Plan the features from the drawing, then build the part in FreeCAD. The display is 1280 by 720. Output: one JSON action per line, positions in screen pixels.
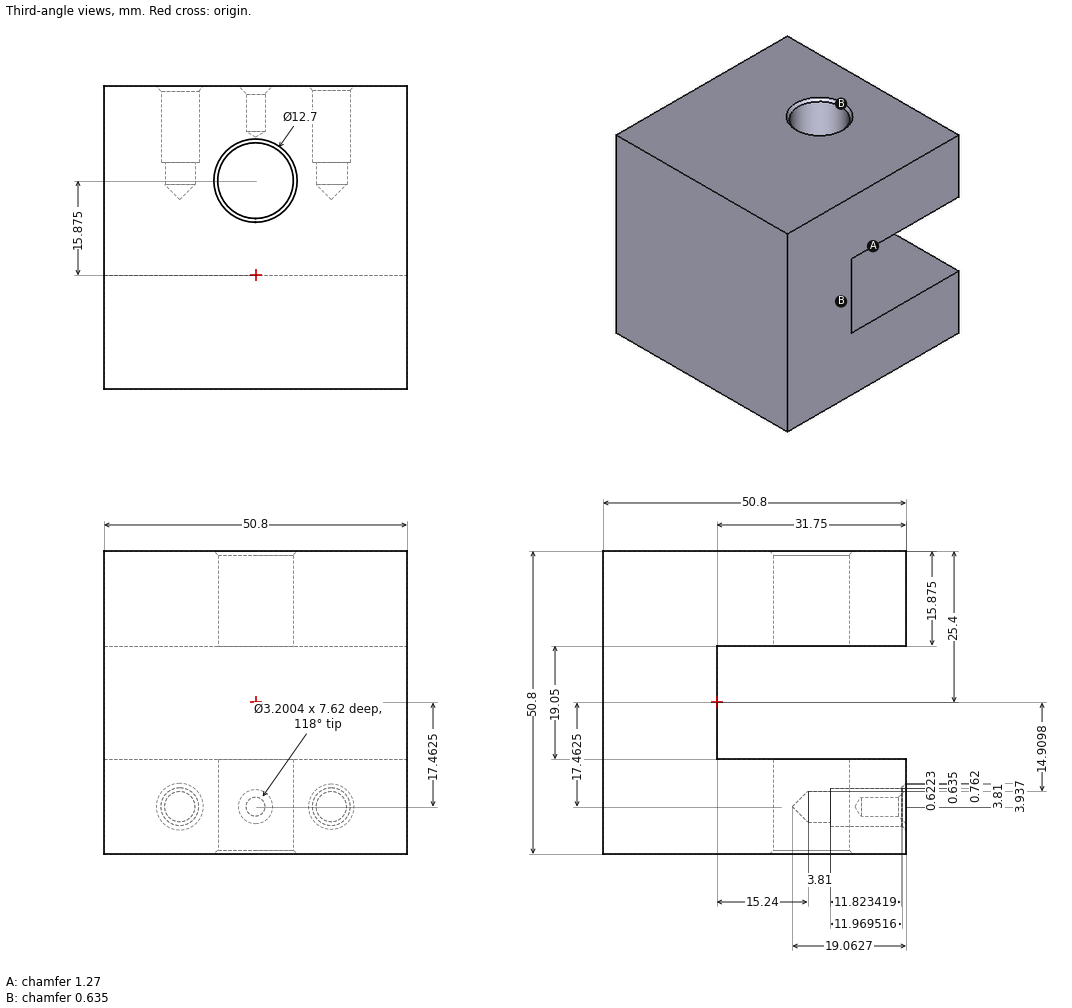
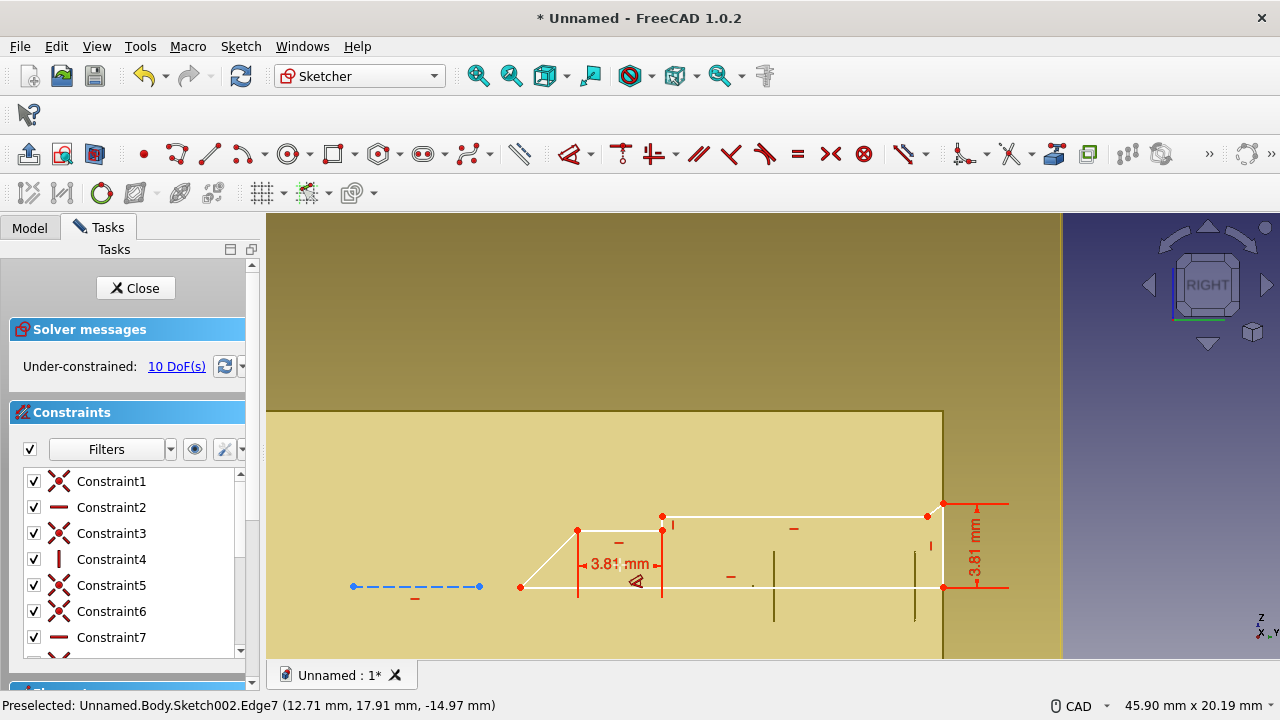
{"action": "scroll", "coordinate": [662, 524], "scroll_direction": "up", "scroll_amount": 6}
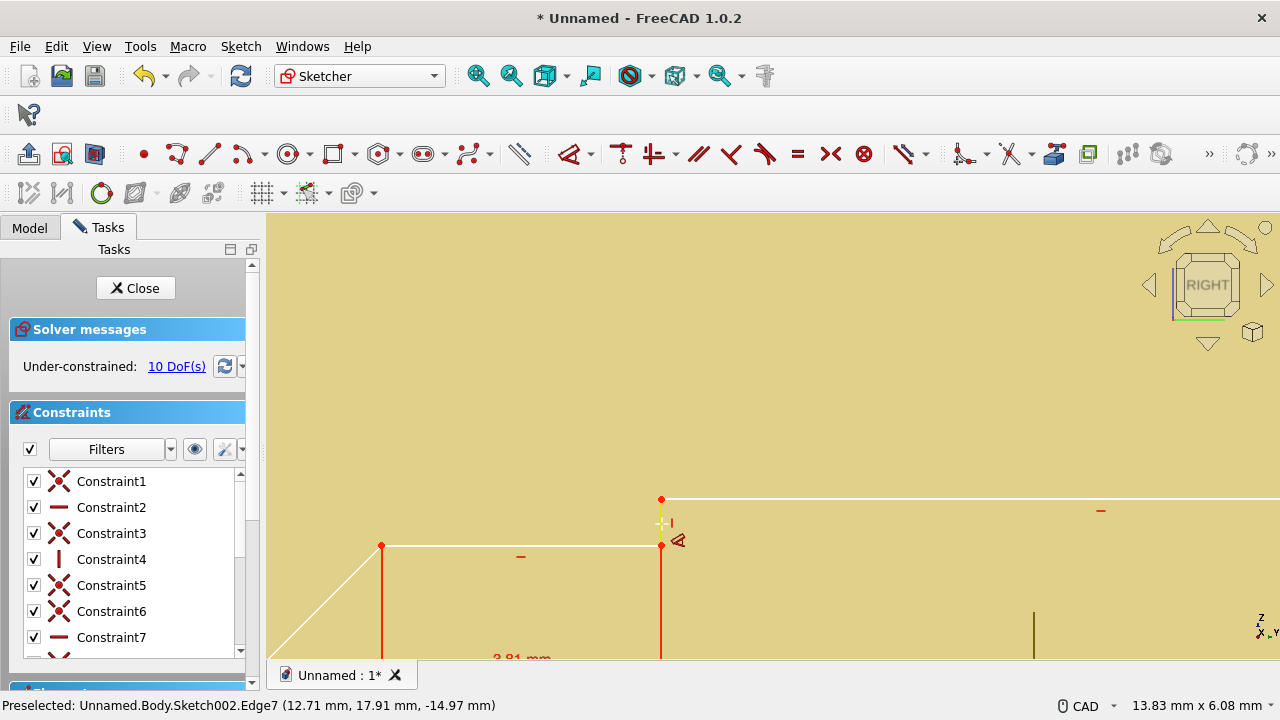
{"action": "left_click", "coordinate": [661, 522]}
{"action": "left_click", "coordinate": [695, 522]}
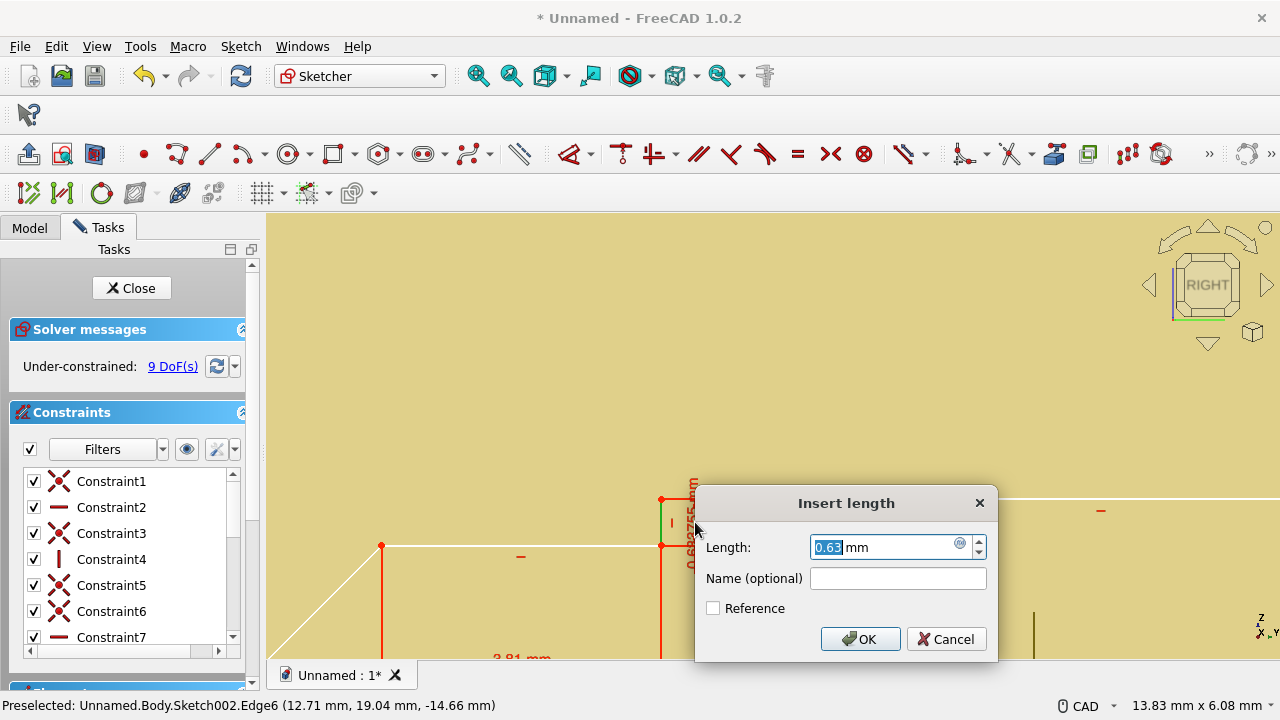
{"action": "type", "text": "0.6223"}
{"action": "key", "text": "Return"}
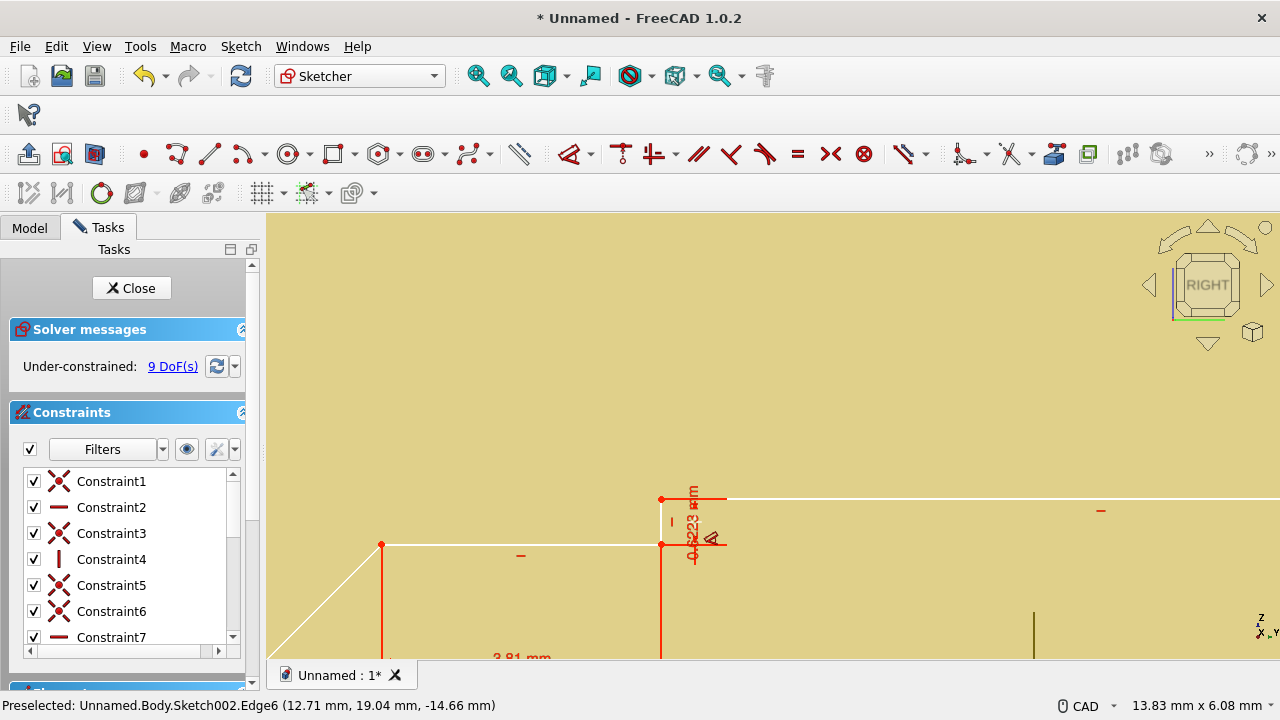
{"action": "scroll", "coordinate": [774, 524], "scroll_direction": "down", "scroll_amount": 8}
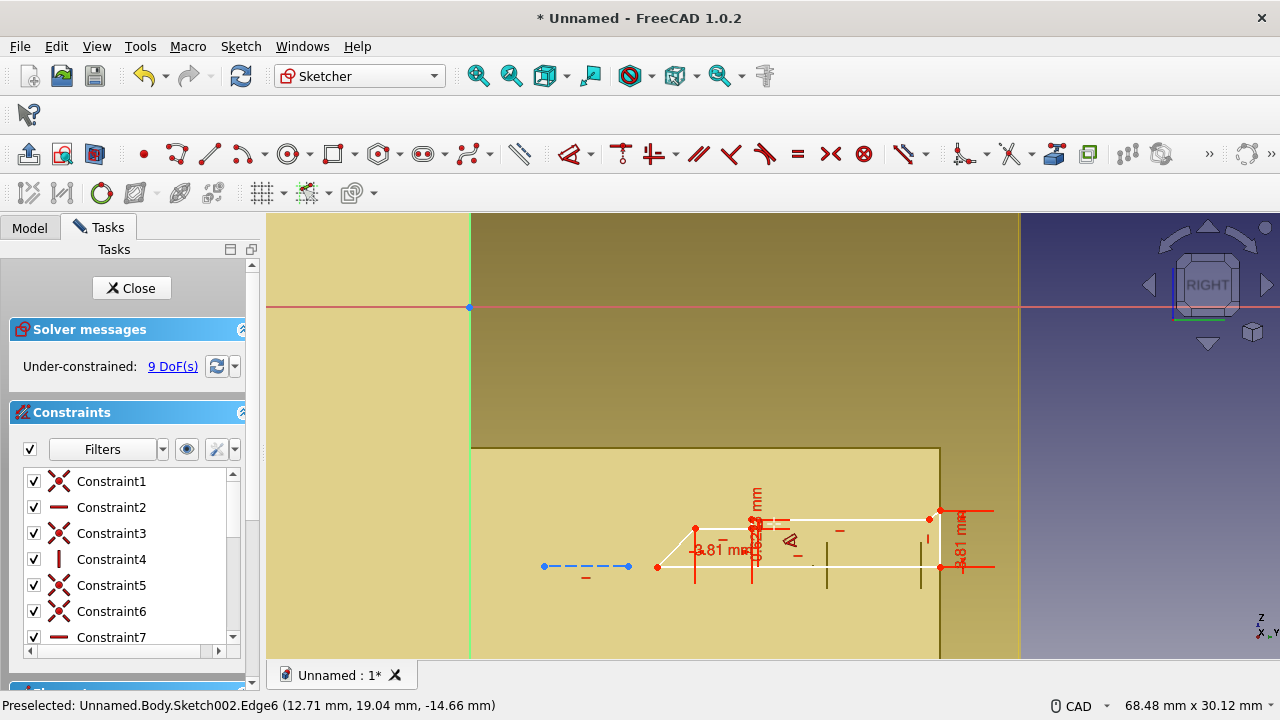
{"action": "left_click", "coordinate": [695, 529]}
{"action": "left_click", "coordinate": [582, 273]}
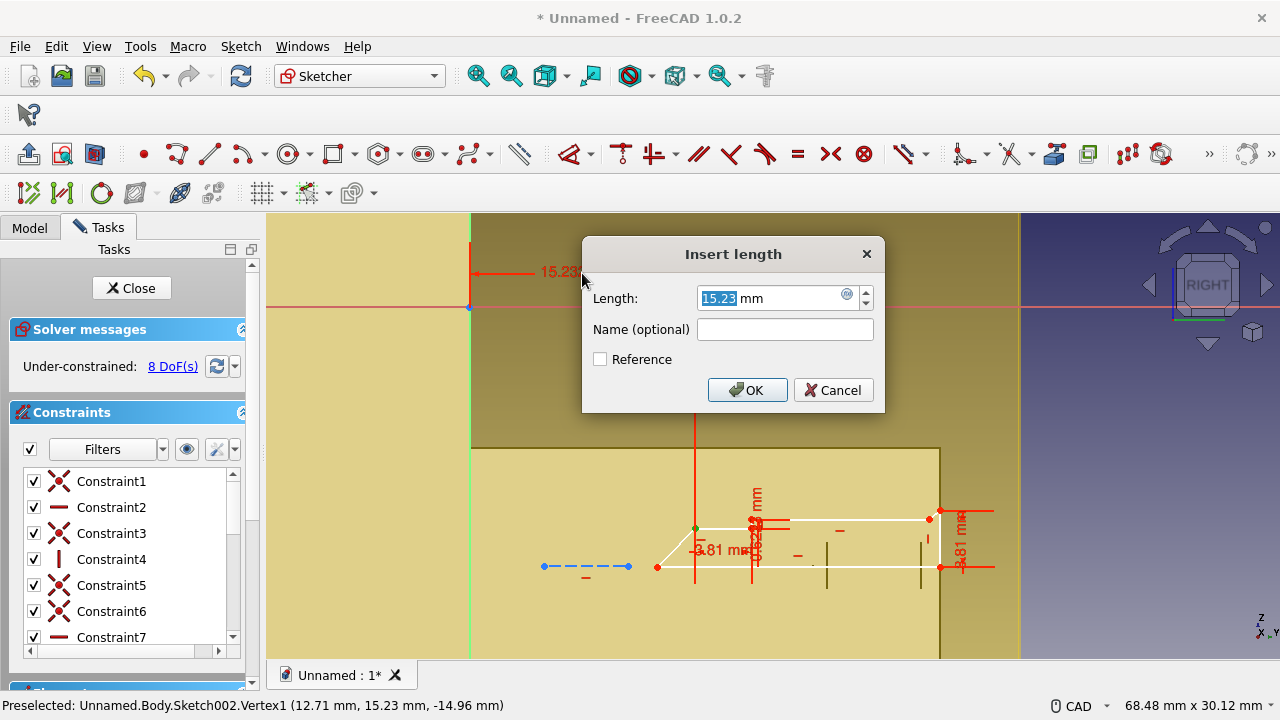
{"action": "type", "text": "15.24"}
{"action": "key", "text": "Return"}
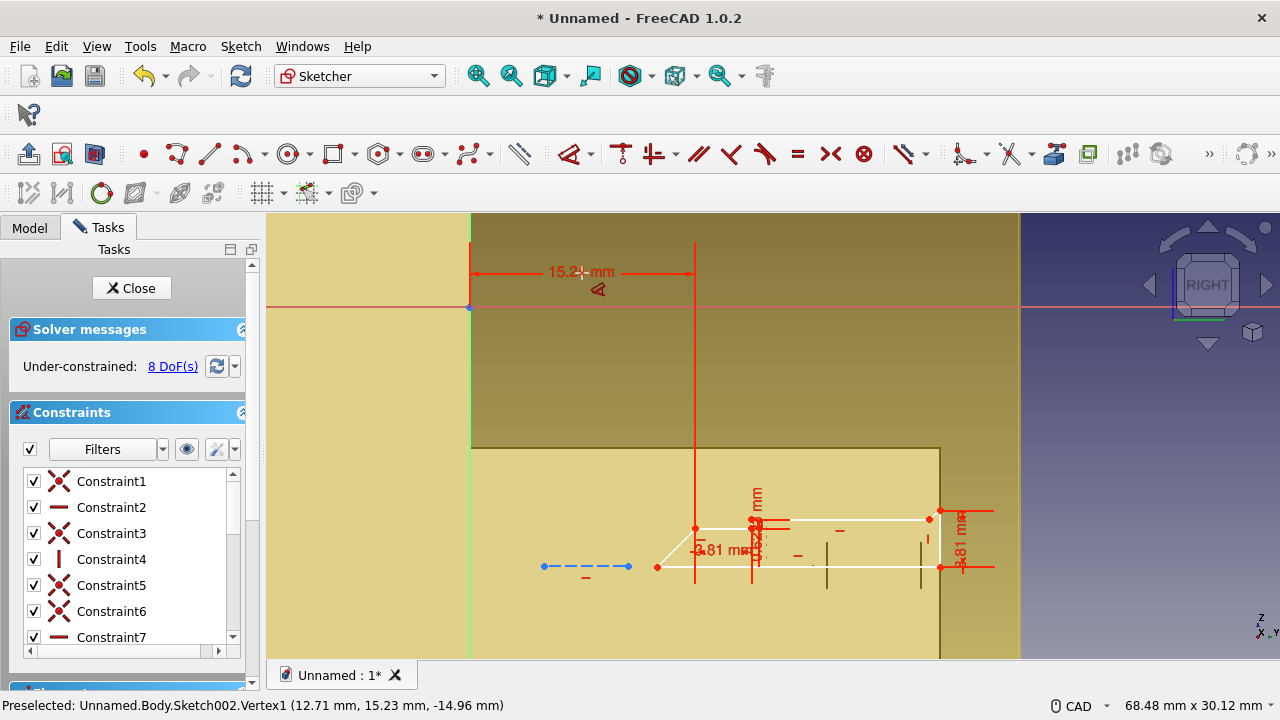
{"action": "left_click", "coordinate": [940, 567]}
{"action": "left_click", "coordinate": [705, 601]}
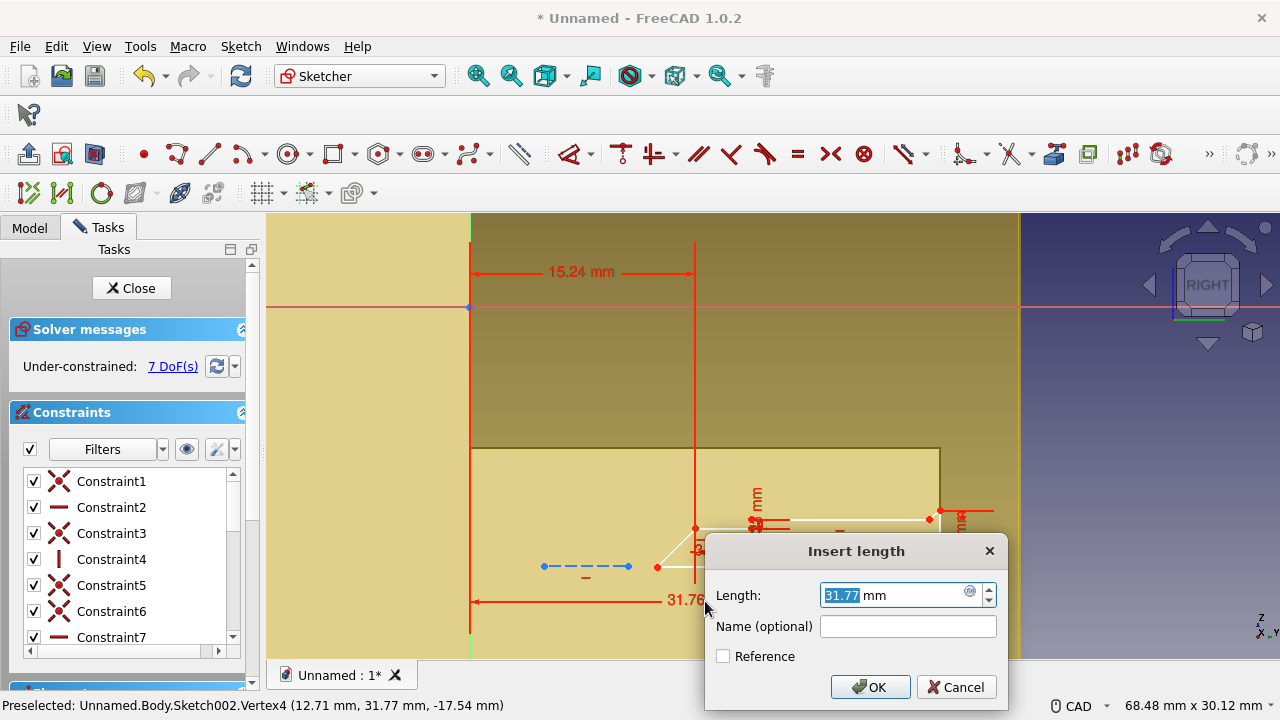
{"action": "type", "text": "31.75"}
{"action": "key", "text": "Return"}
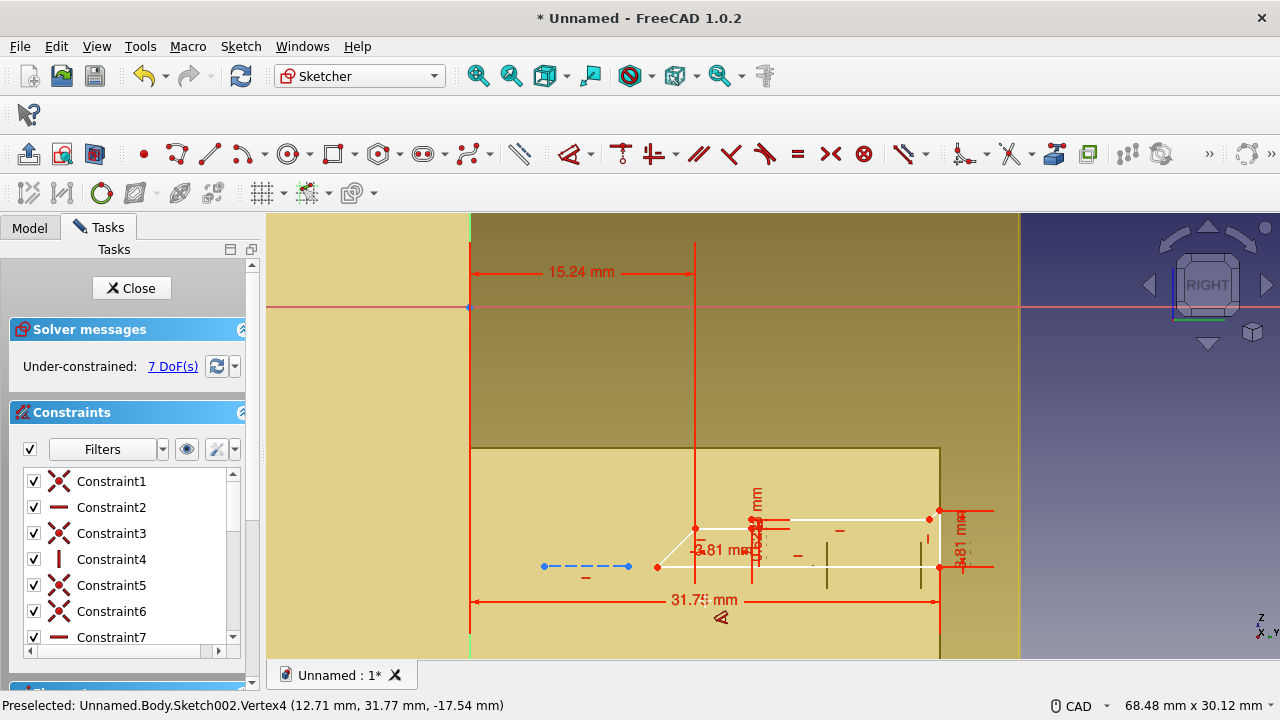
{"action": "scroll", "coordinate": [933, 516], "scroll_direction": "up", "scroll_amount": 8}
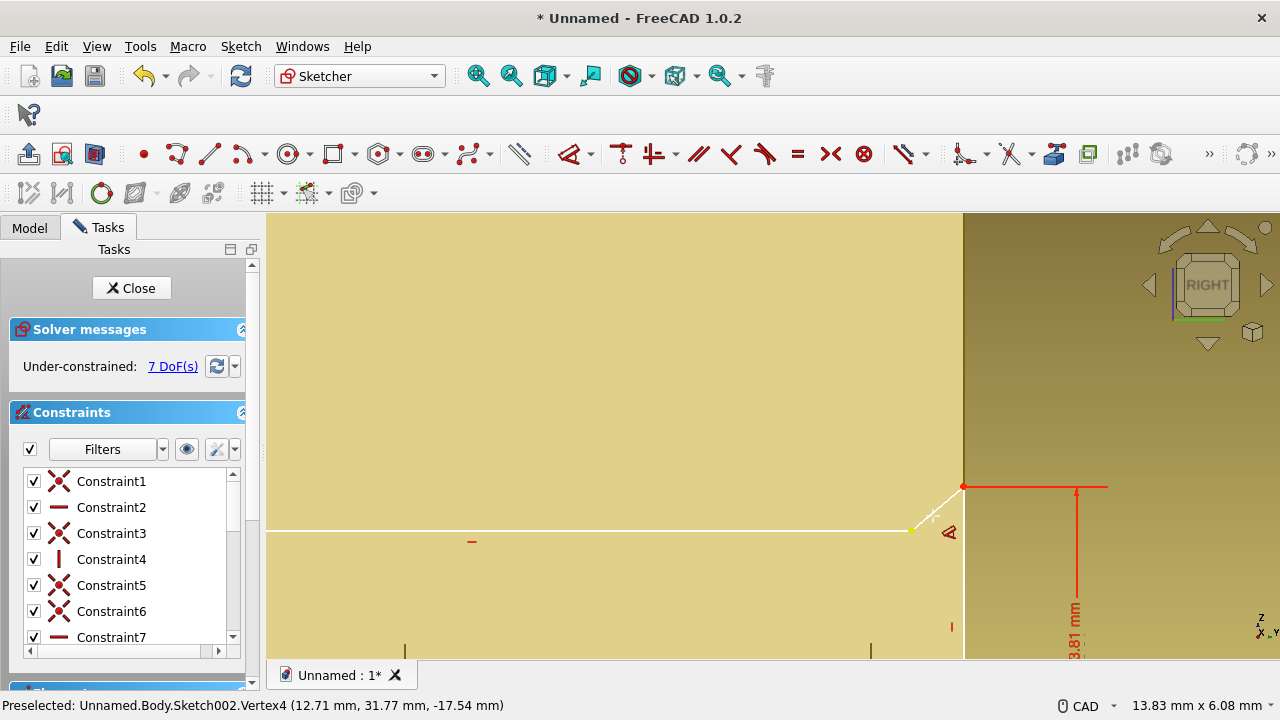
{"action": "left_click", "coordinate": [933, 513]}
{"action": "left_click", "coordinate": [998, 509]}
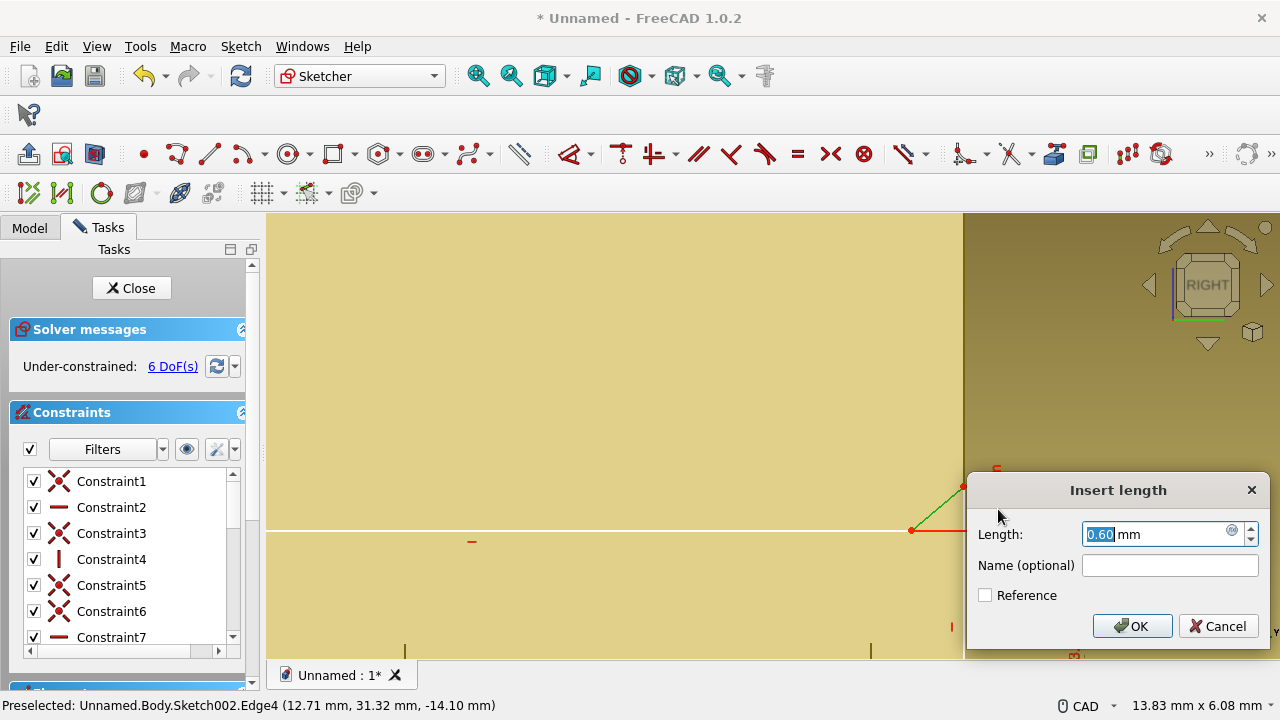
{"action": "type", "text": "0.635"}
{"action": "key", "text": "Return"}